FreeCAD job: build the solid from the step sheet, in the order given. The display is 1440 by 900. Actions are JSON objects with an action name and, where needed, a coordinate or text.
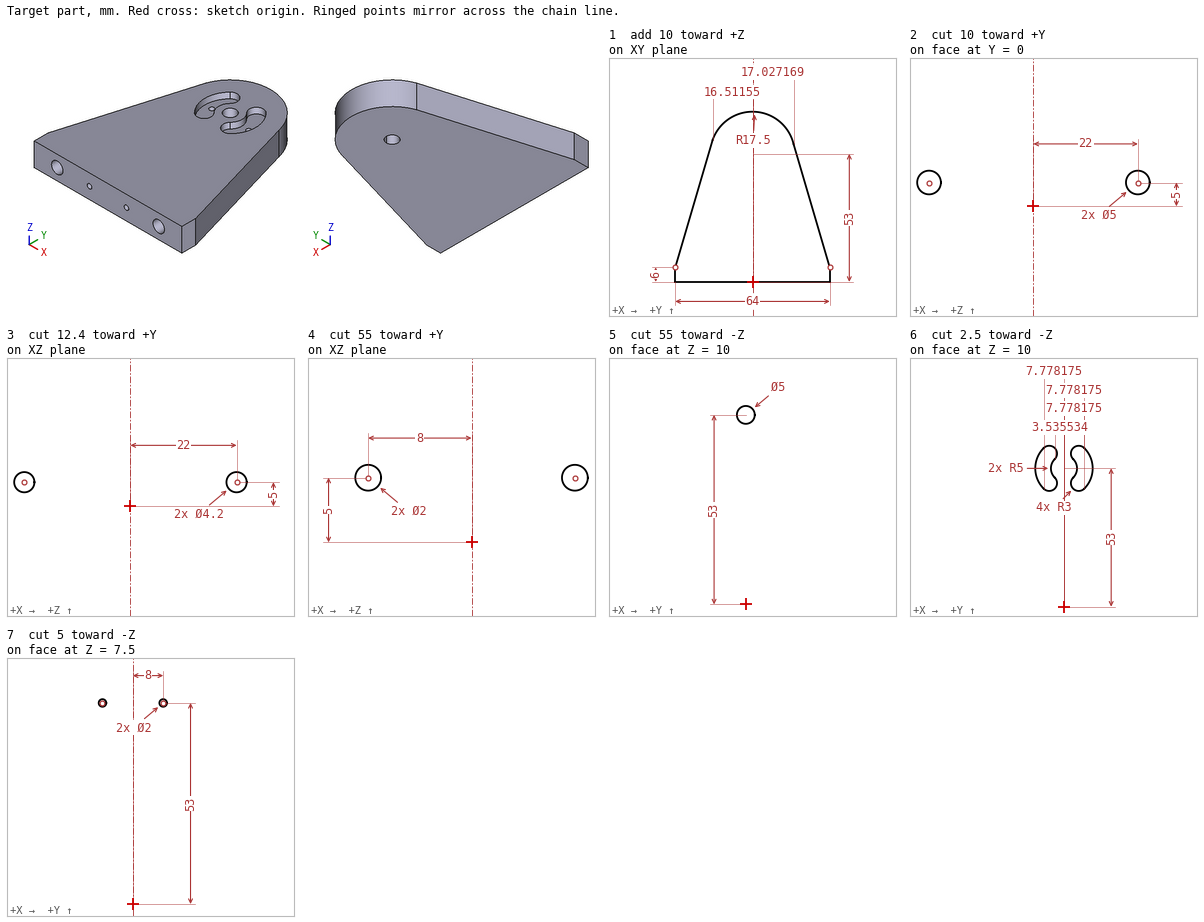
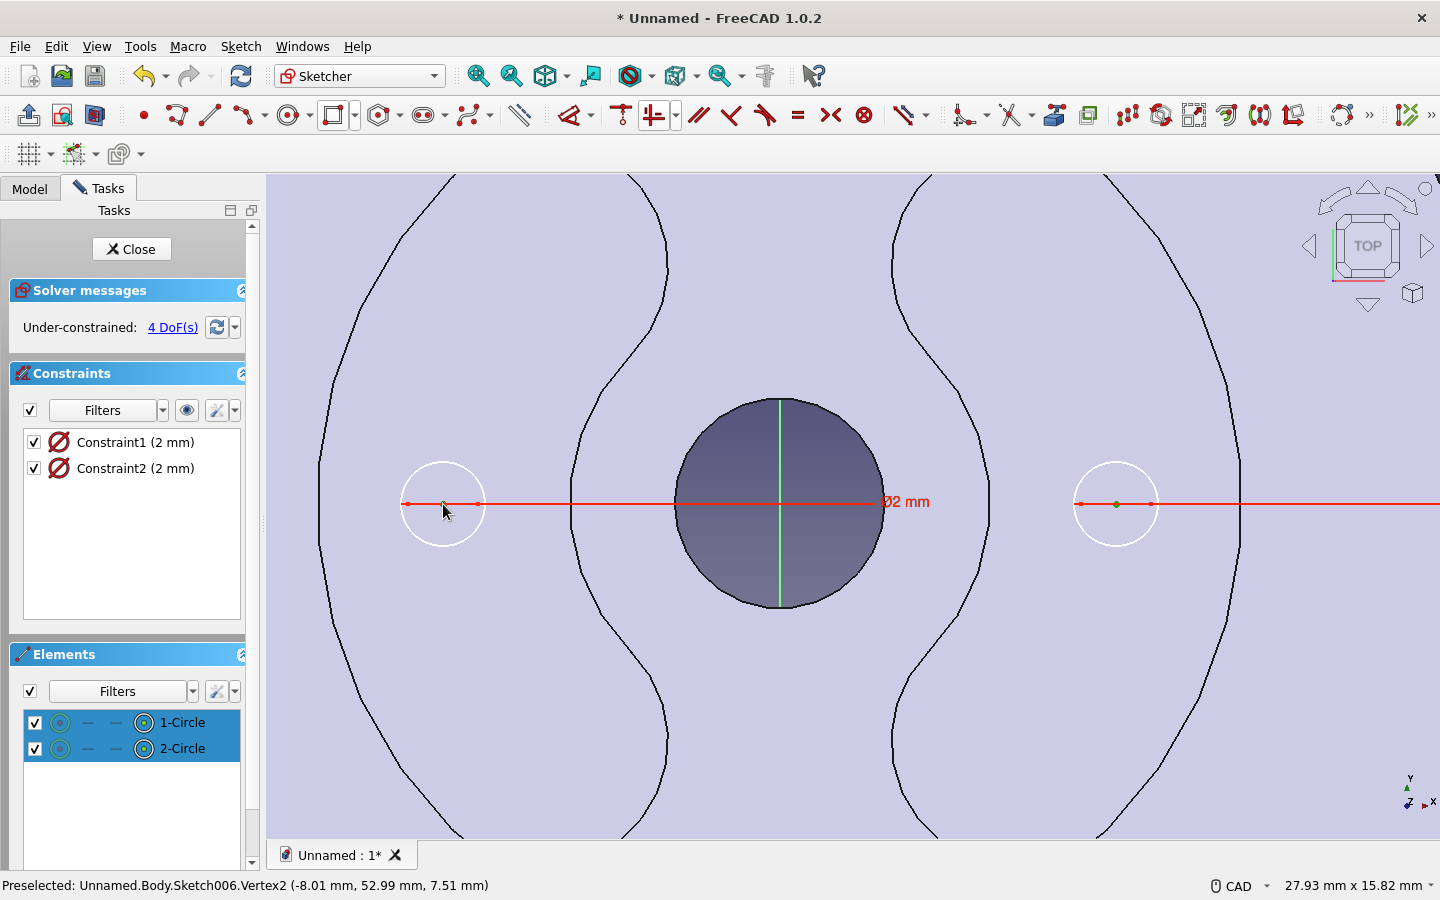
{"action": "left_click", "coordinate": [780, 768]}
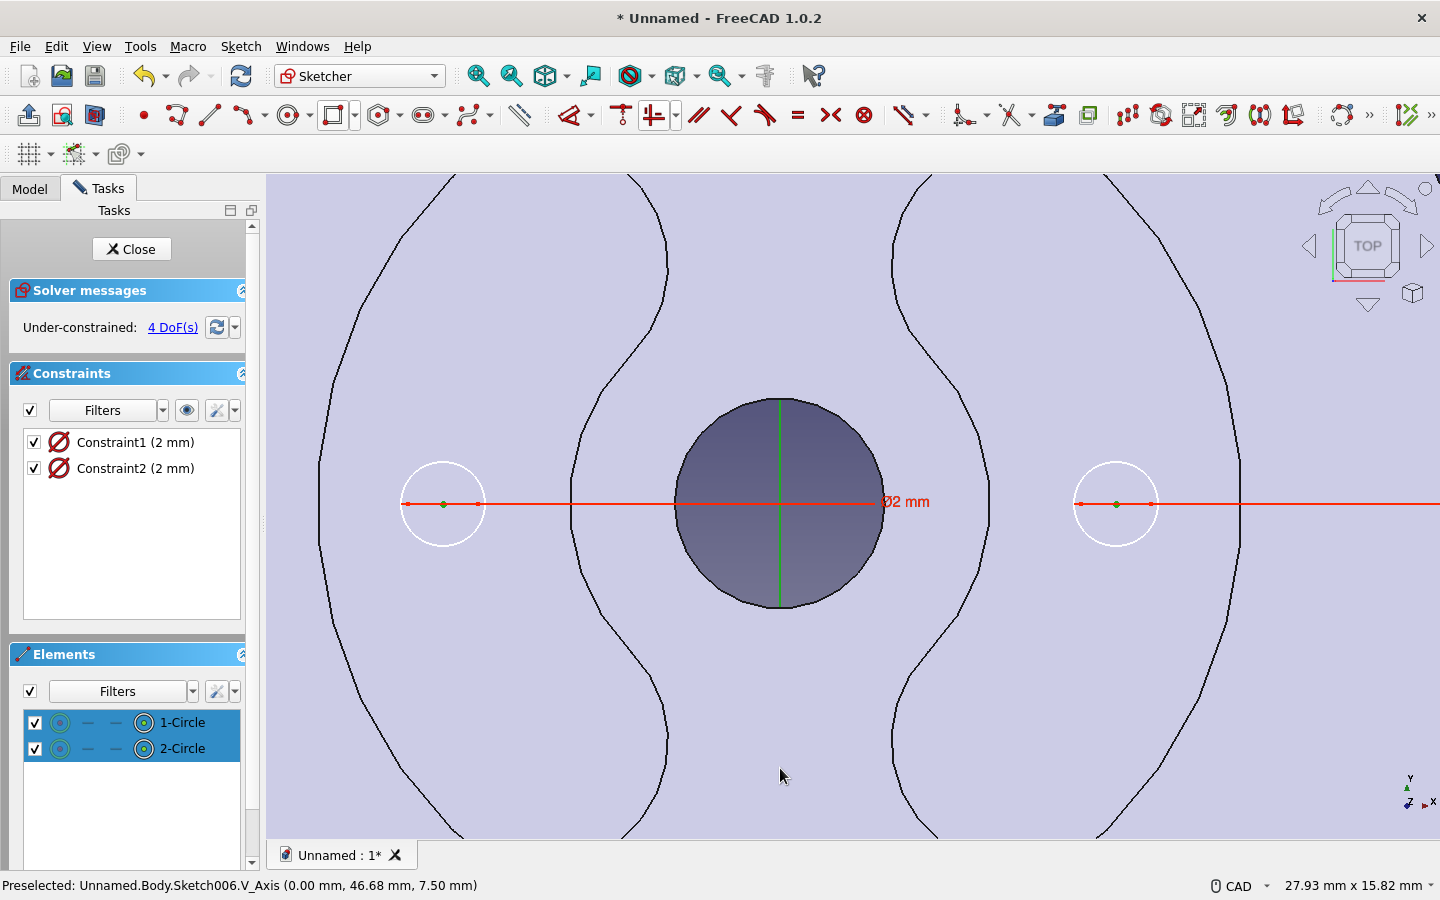
{"action": "left_click", "coordinate": [831, 116]}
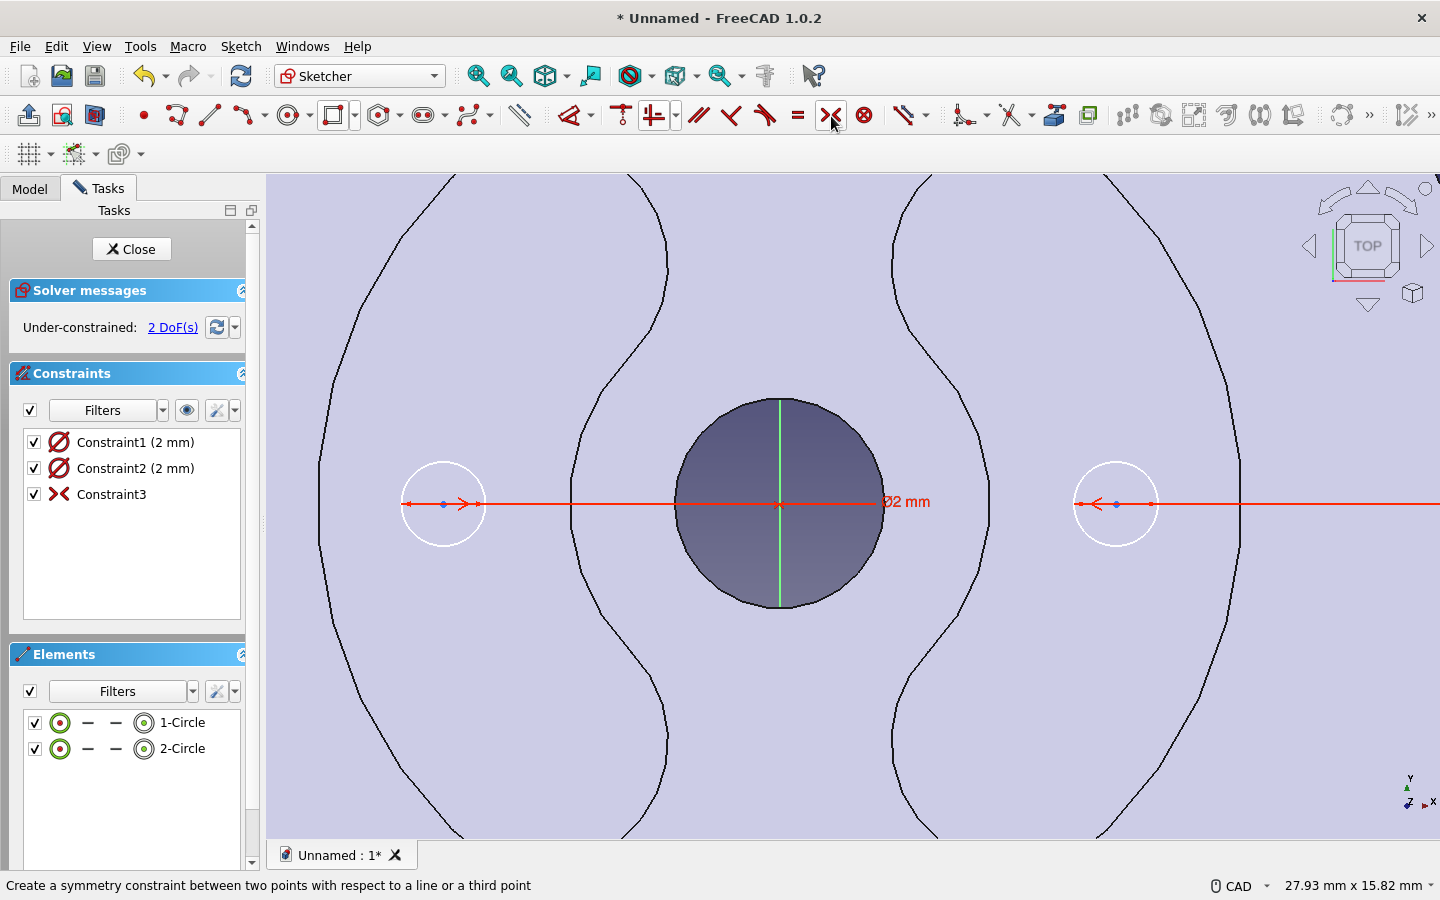
{"action": "left_click", "coordinate": [568, 116]}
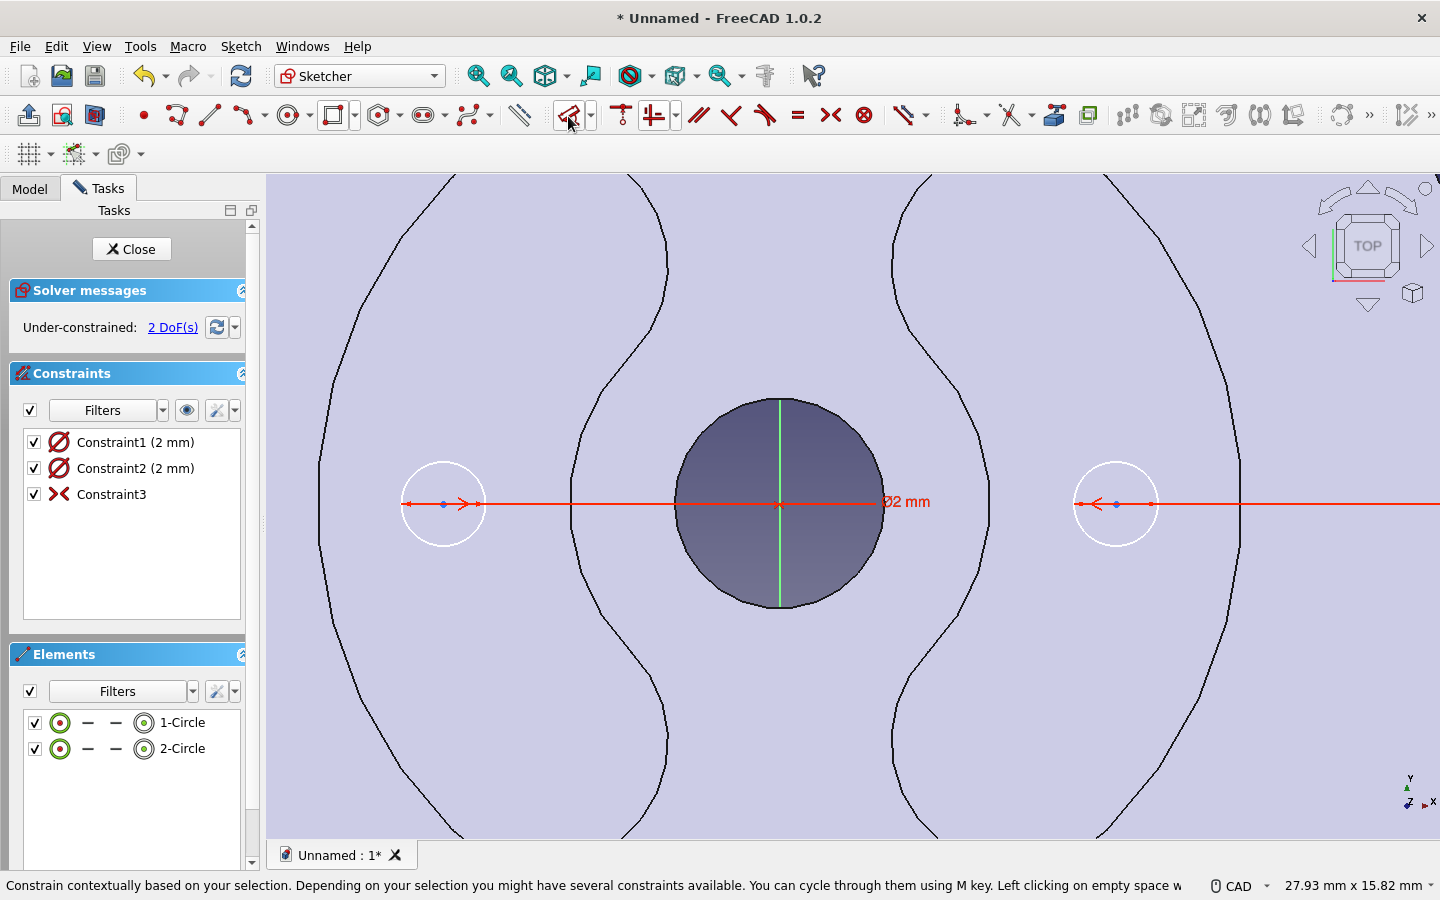
{"action": "left_click", "coordinate": [1116, 504]}
{"action": "left_click", "coordinate": [948, 470]}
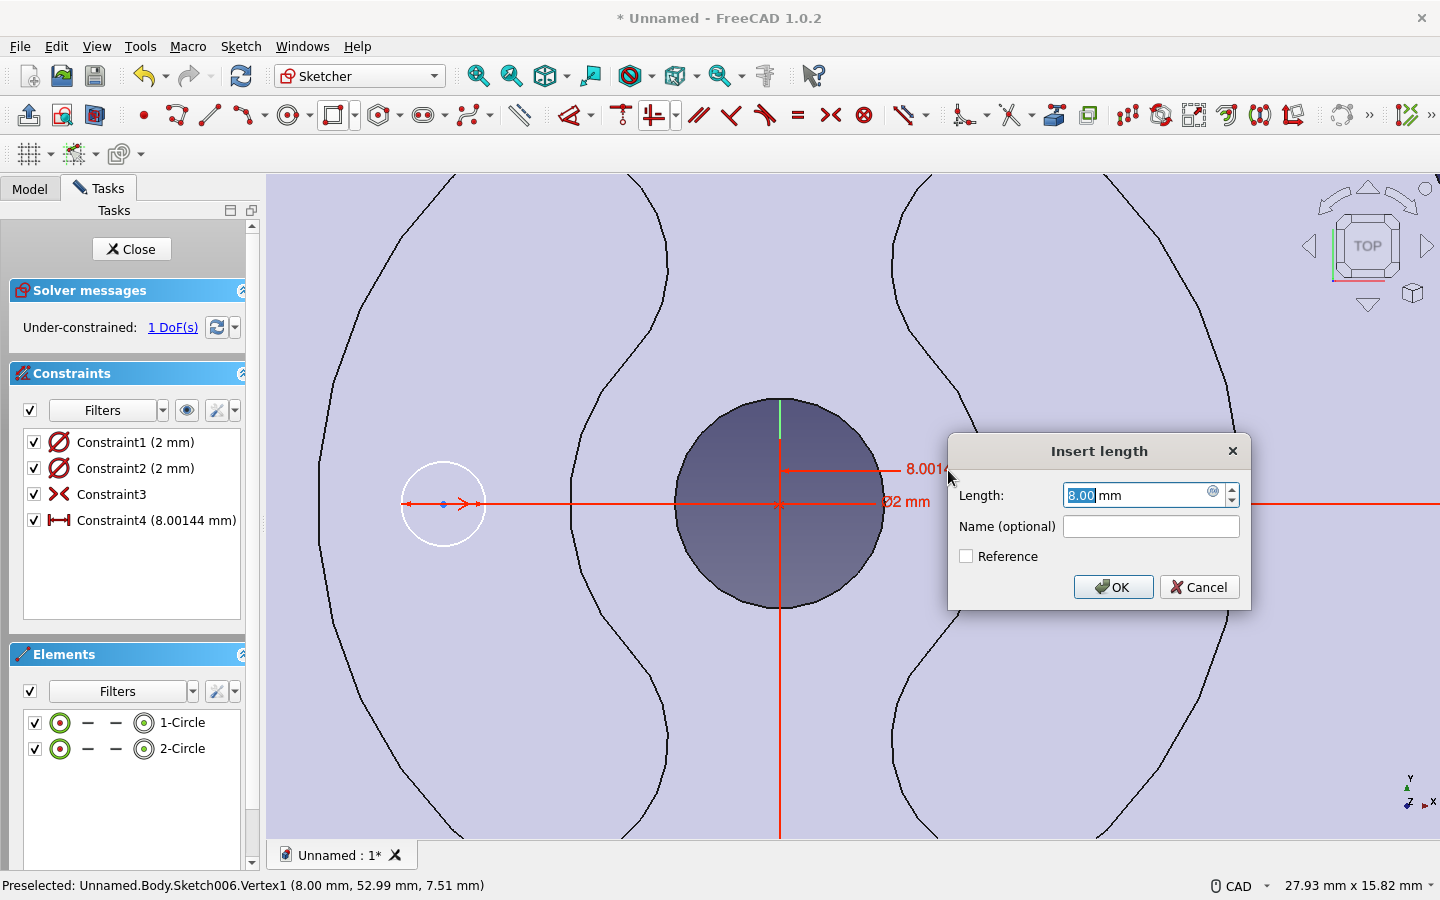
{"action": "type", "text": "8"}
{"action": "key", "text": "Return"}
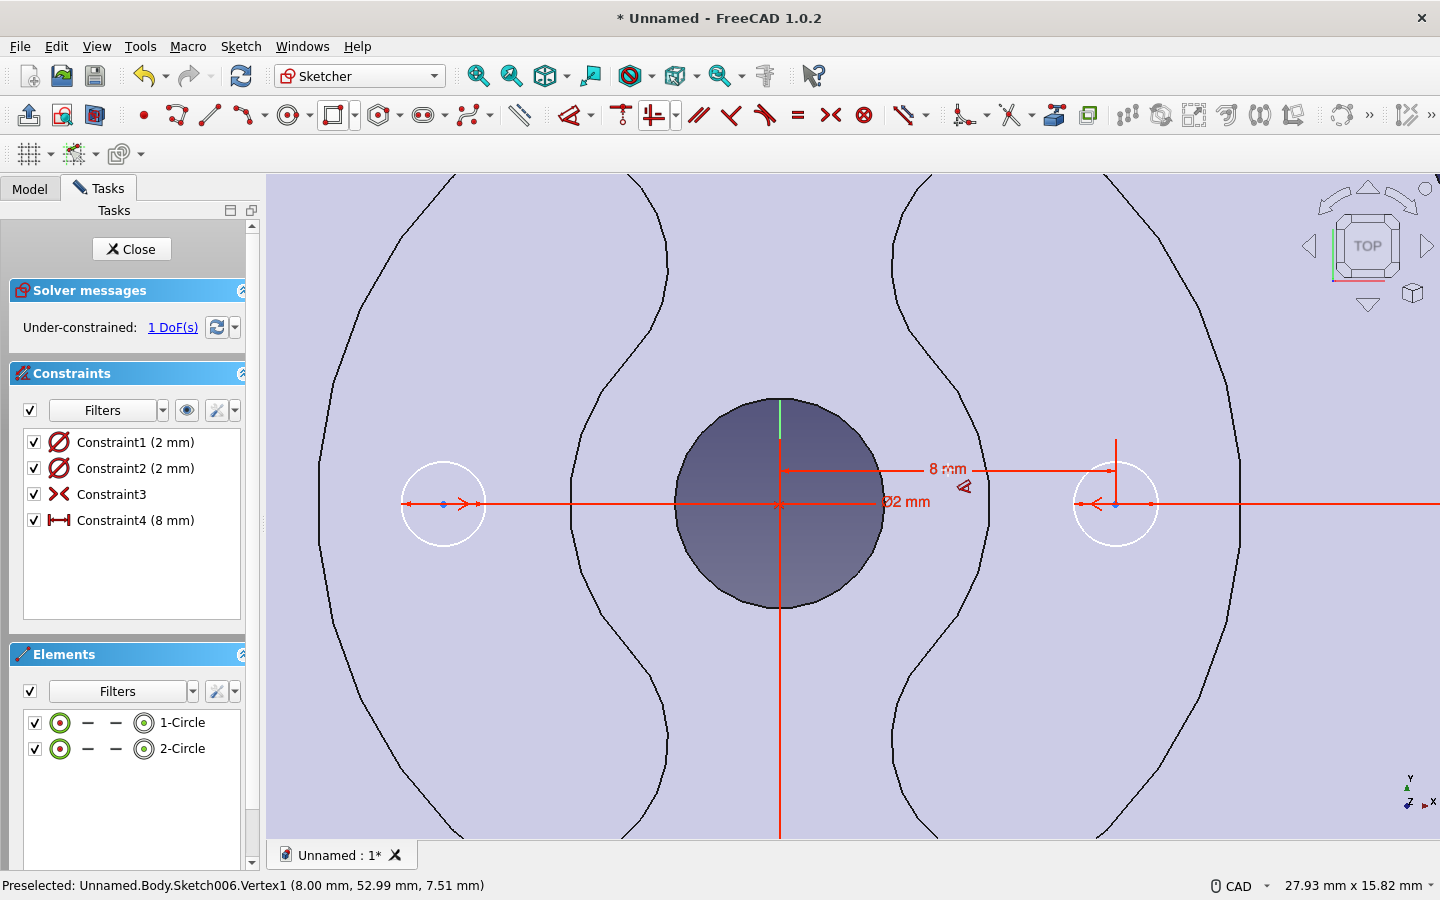
{"action": "left_click", "coordinate": [1116, 504]}
{"action": "left_click", "coordinate": [1150, 658]}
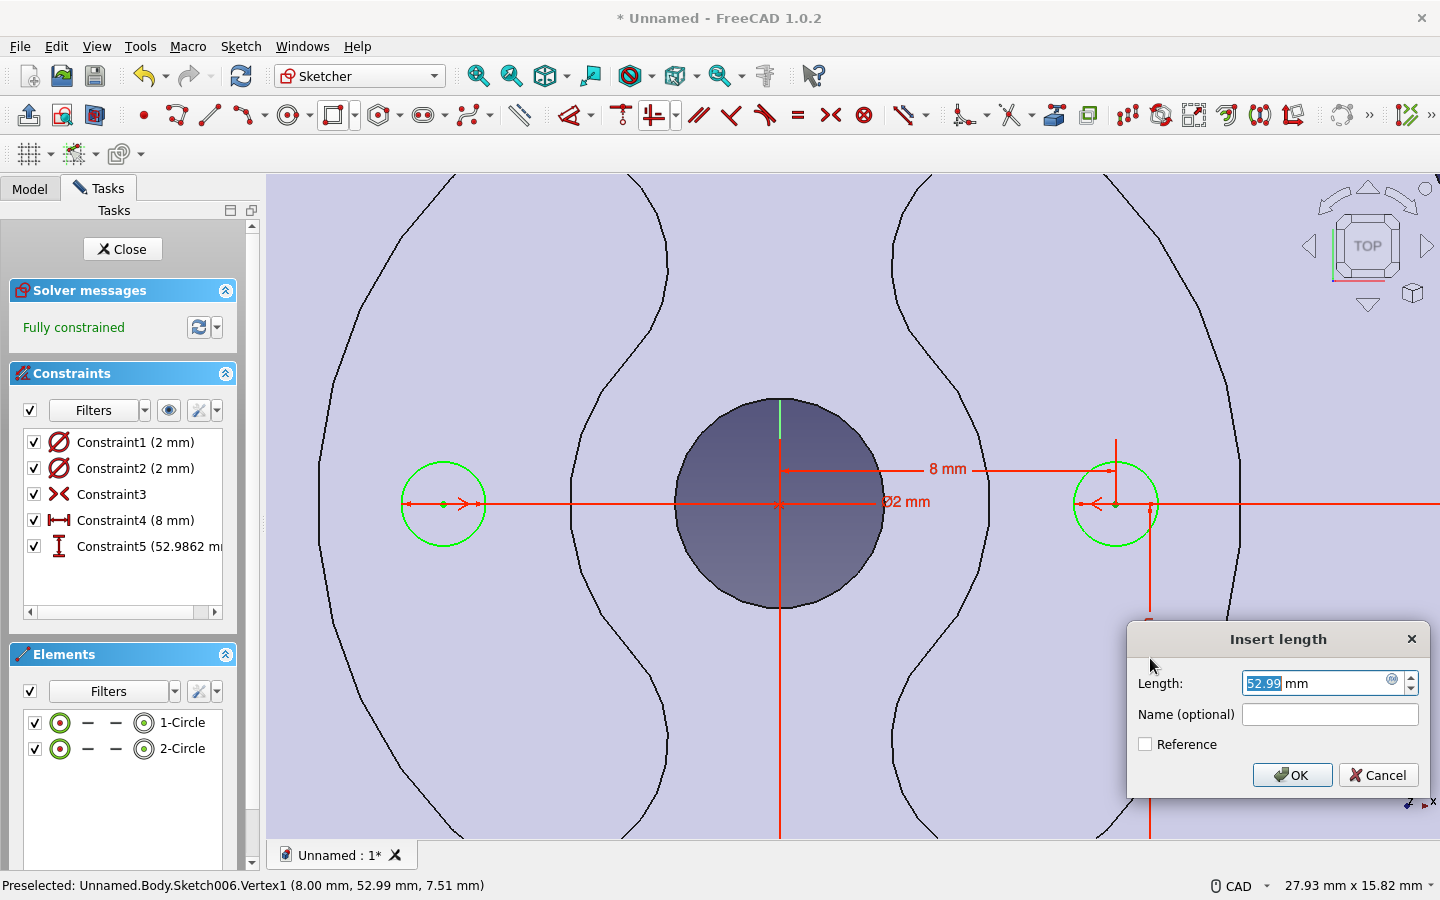
{"action": "type", "text": "53"}
{"action": "key", "text": "Return"}
{"action": "key", "text": "Escape"}